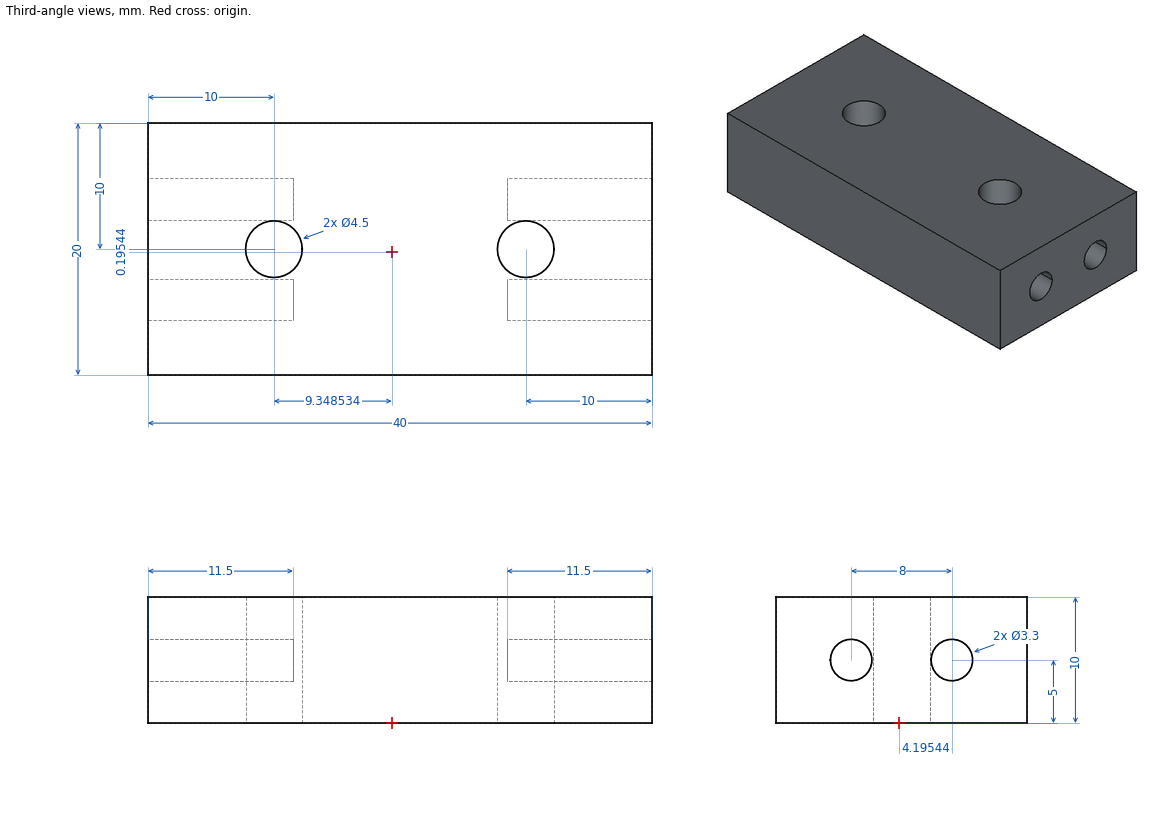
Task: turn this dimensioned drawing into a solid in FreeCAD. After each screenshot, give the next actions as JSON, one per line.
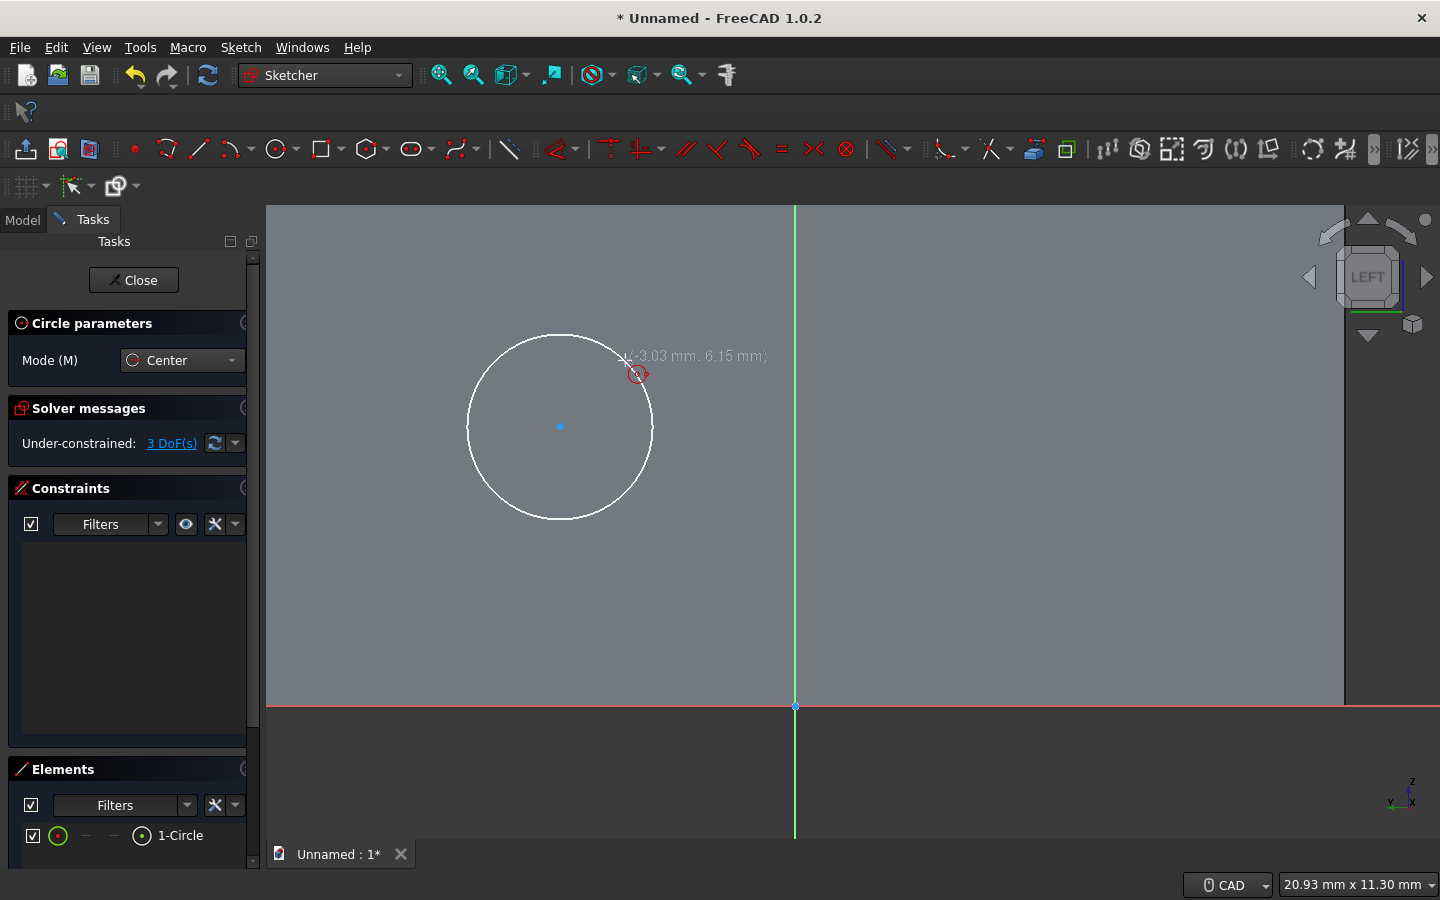
{"action": "left_click", "coordinate": [1009, 426]}
{"action": "left_click", "coordinate": [1074, 360]}
{"action": "key", "text": "Escape"}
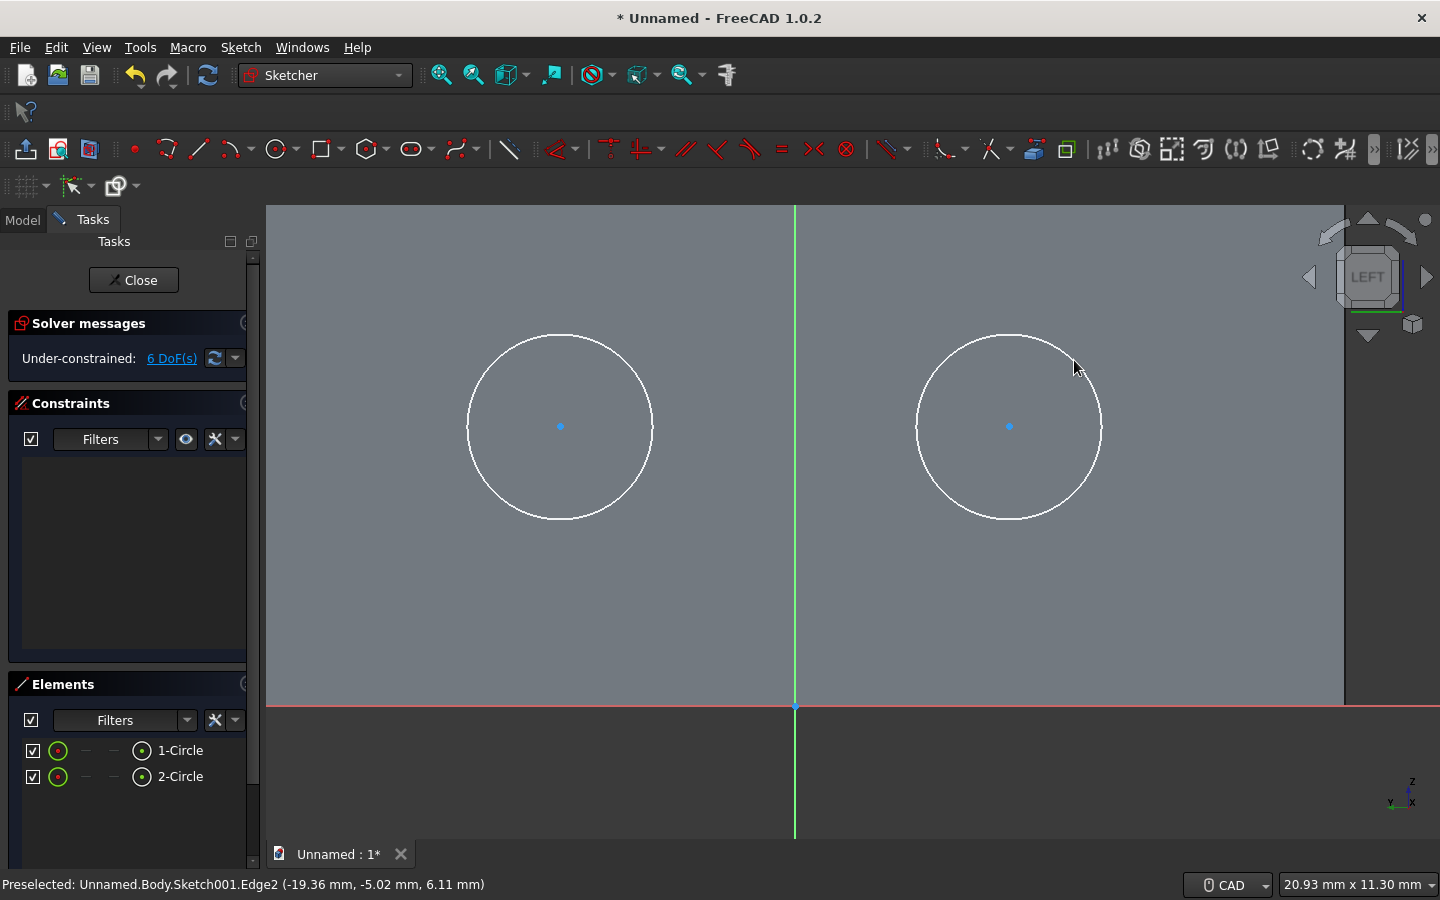
{"action": "left_click", "coordinate": [625, 361]}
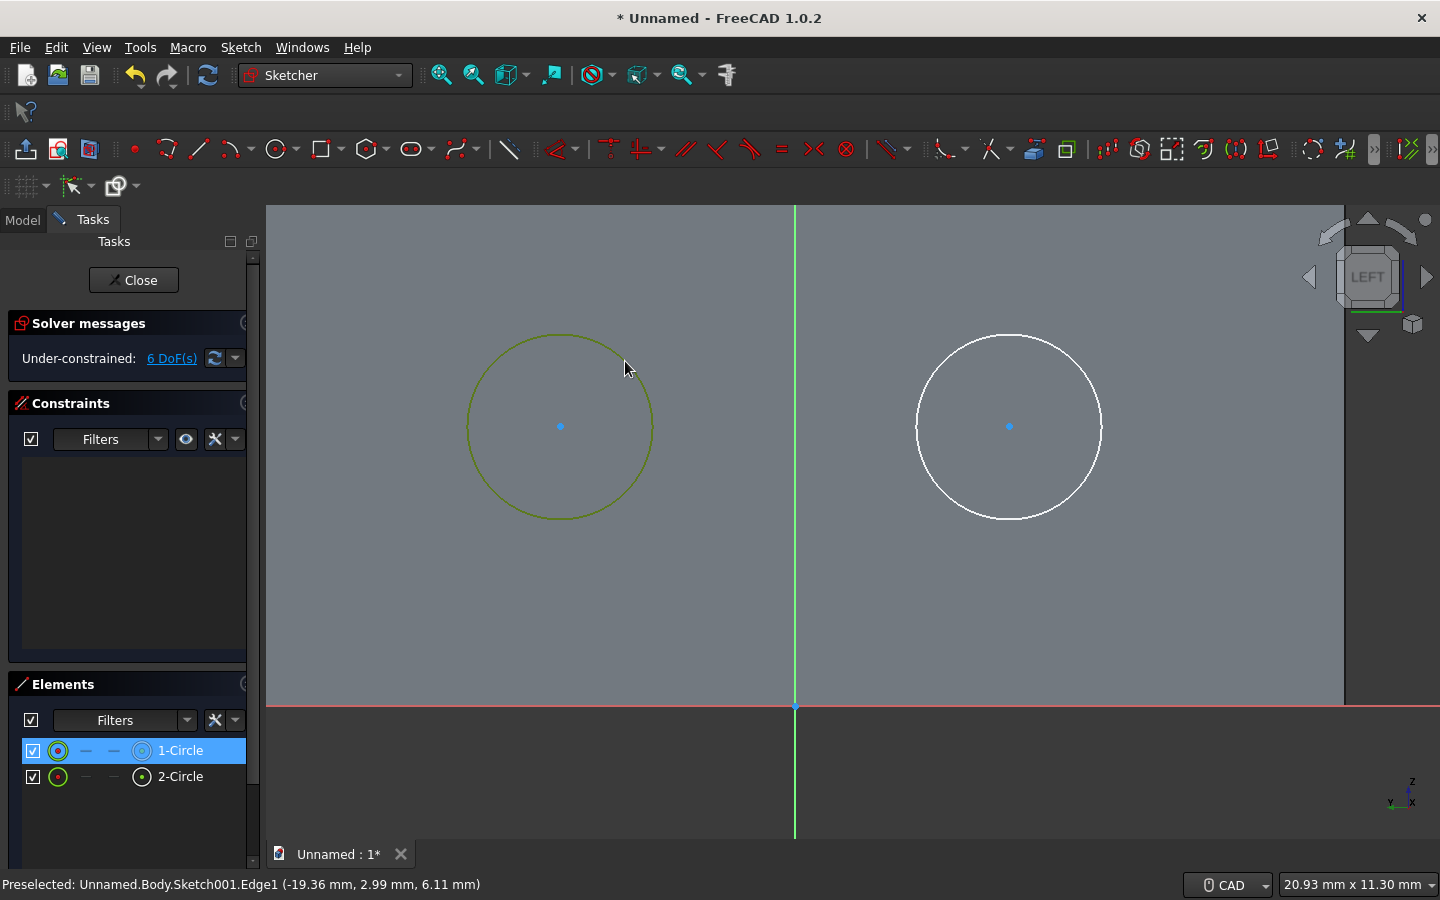
{"action": "left_click", "coordinate": [1074, 361]}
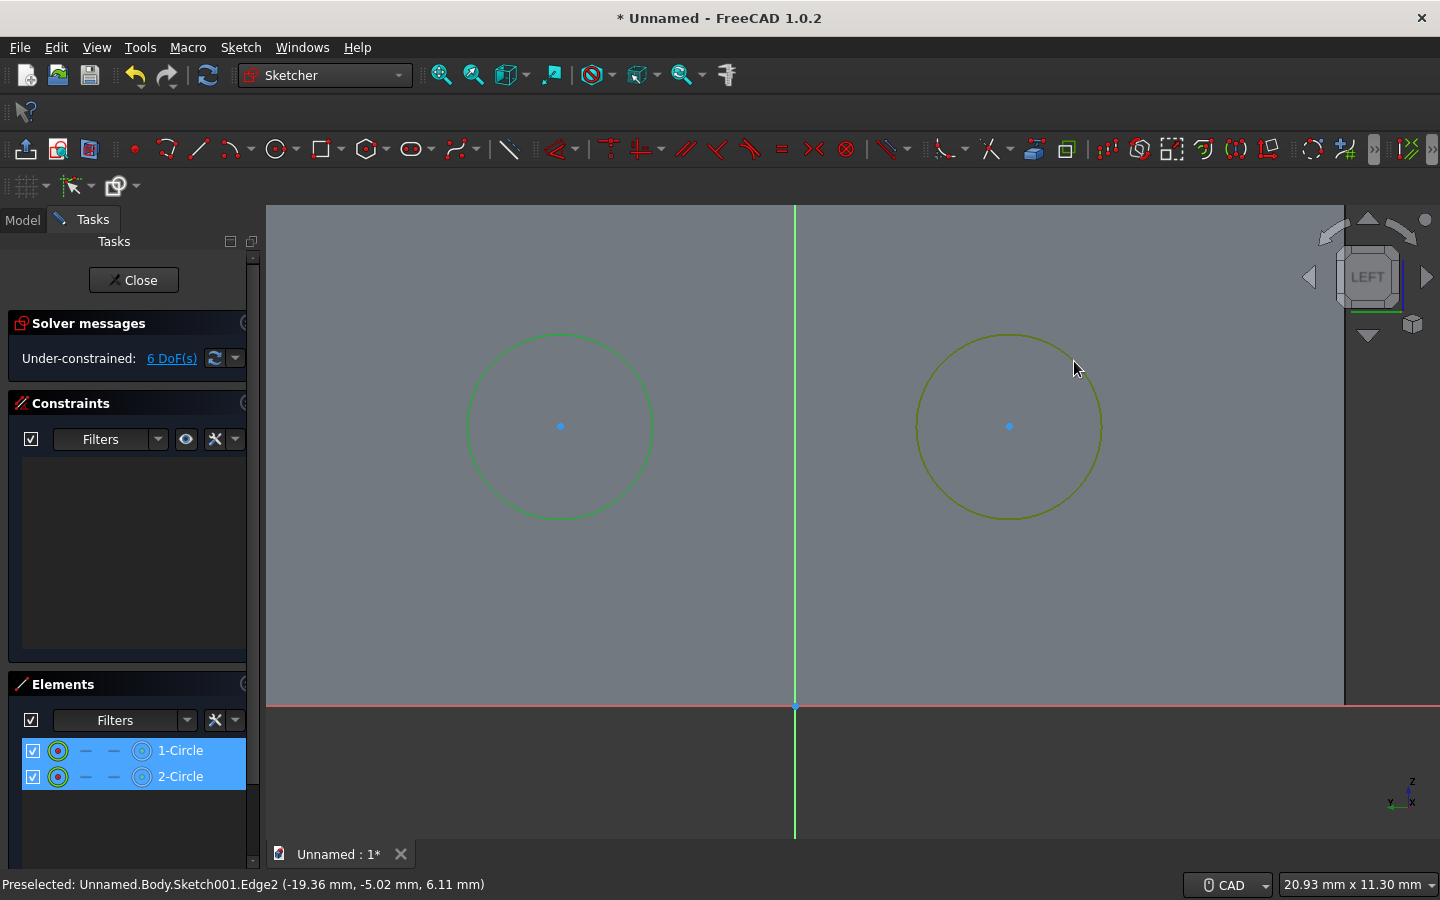
{"action": "key", "text": "e"}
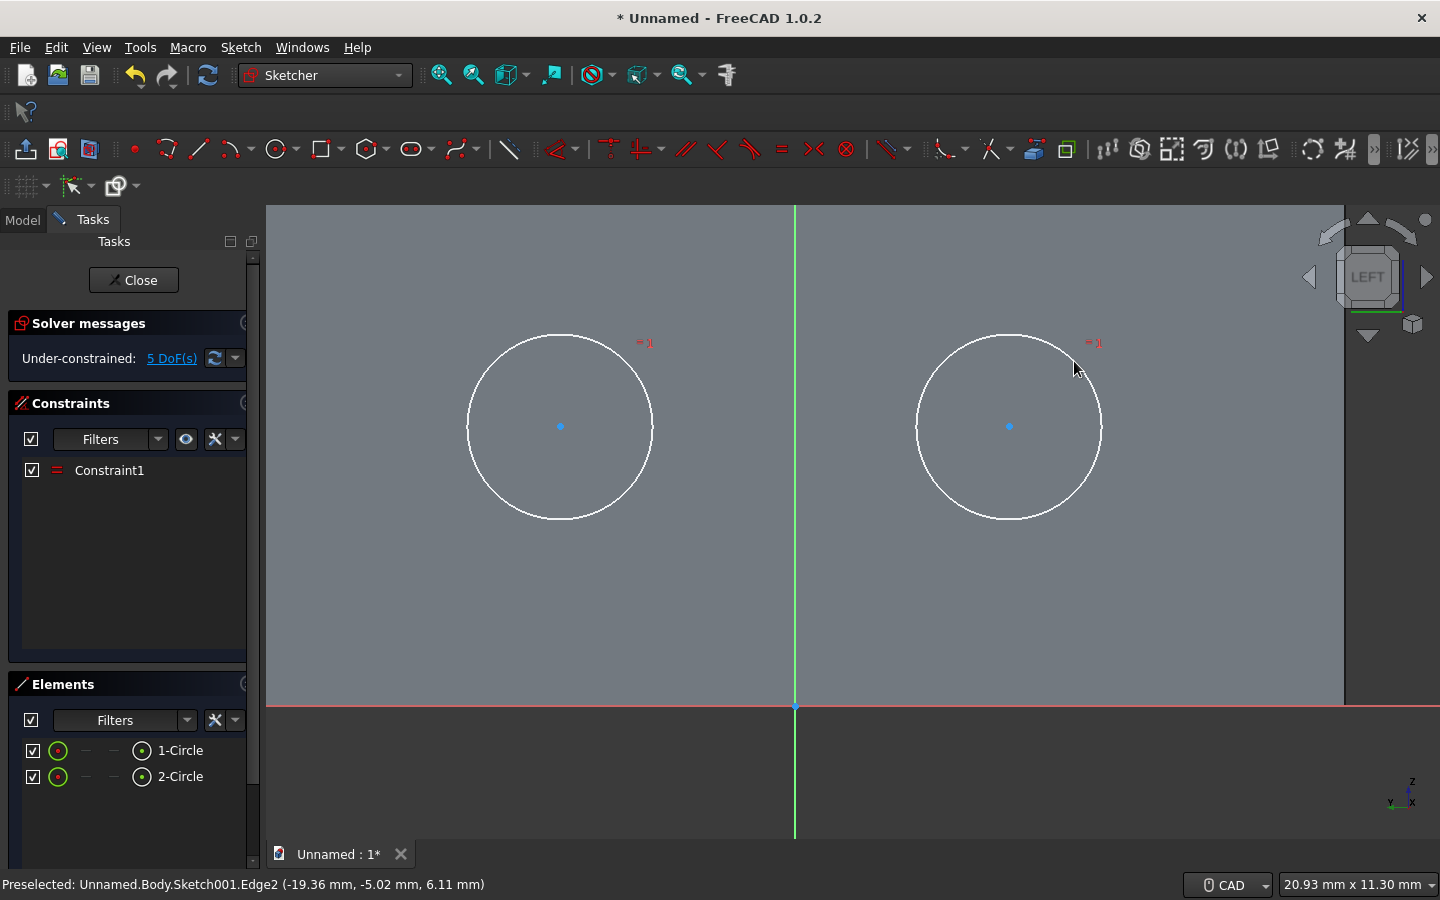
{"action": "left_click", "coordinate": [560, 427]}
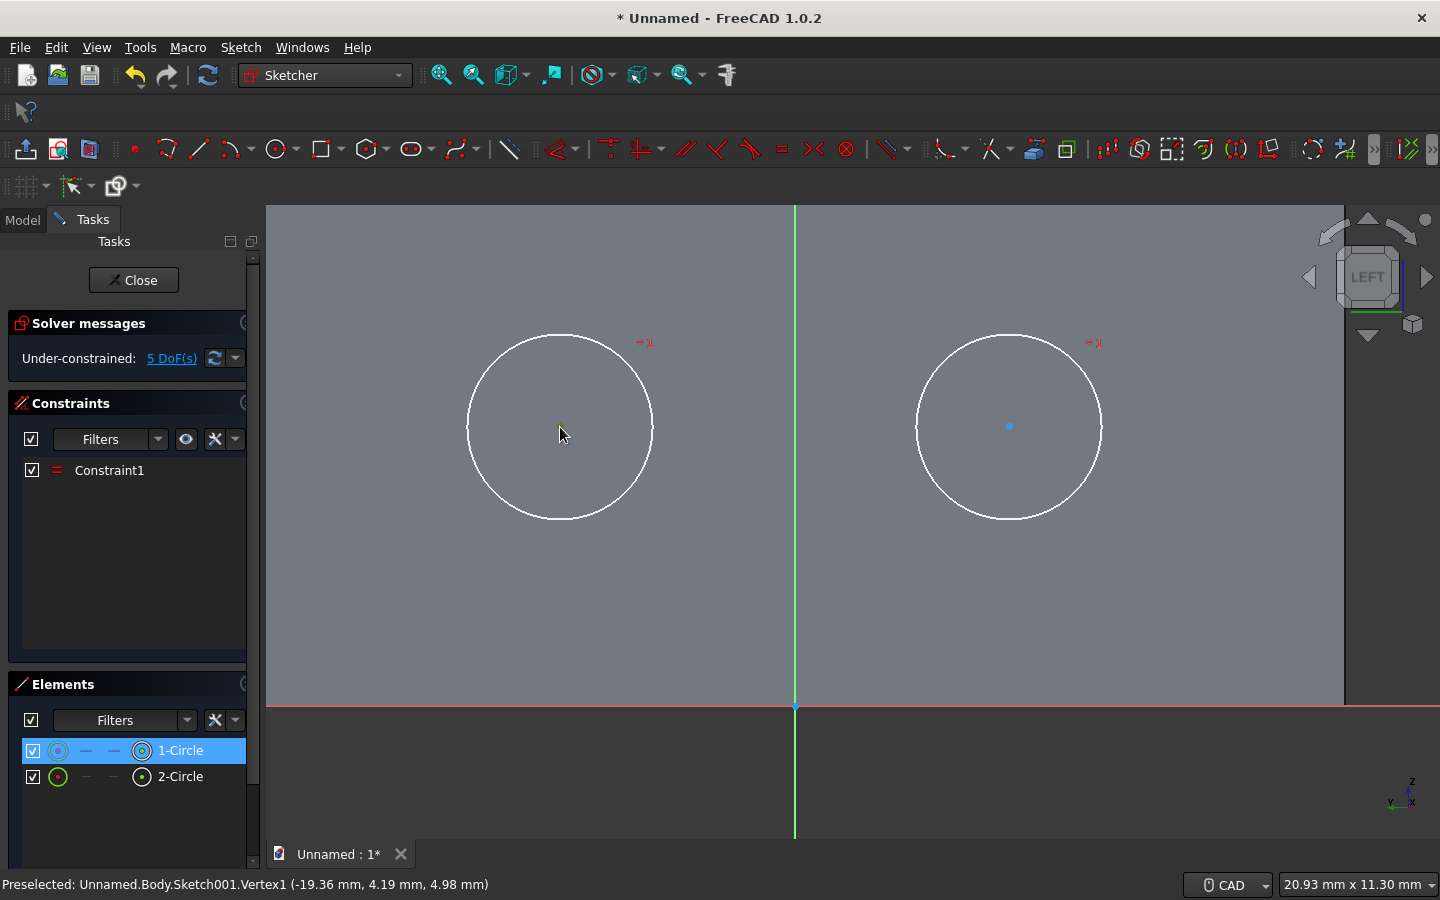
{"action": "left_click", "coordinate": [1009, 427]}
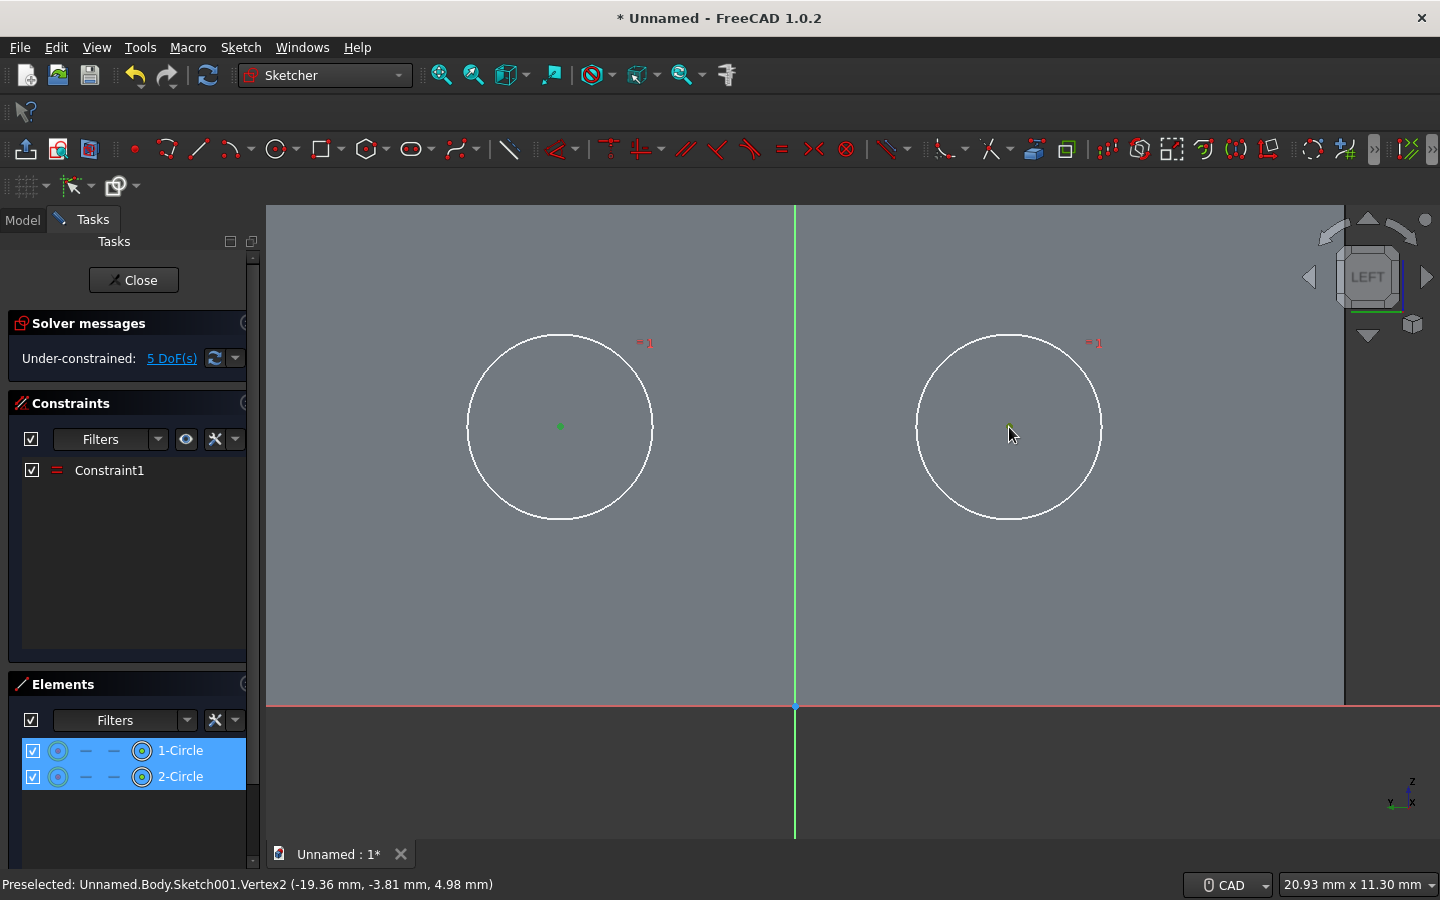
{"action": "key", "text": "h"}